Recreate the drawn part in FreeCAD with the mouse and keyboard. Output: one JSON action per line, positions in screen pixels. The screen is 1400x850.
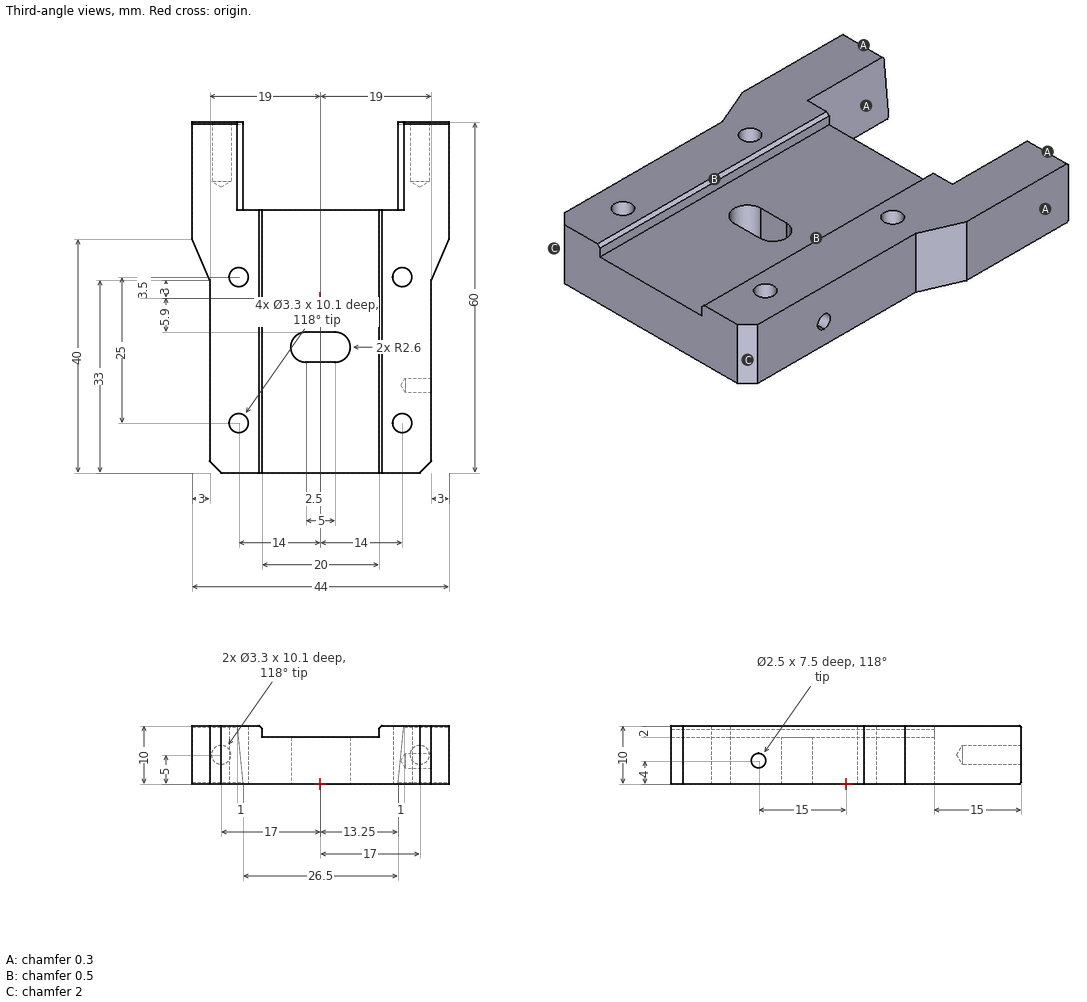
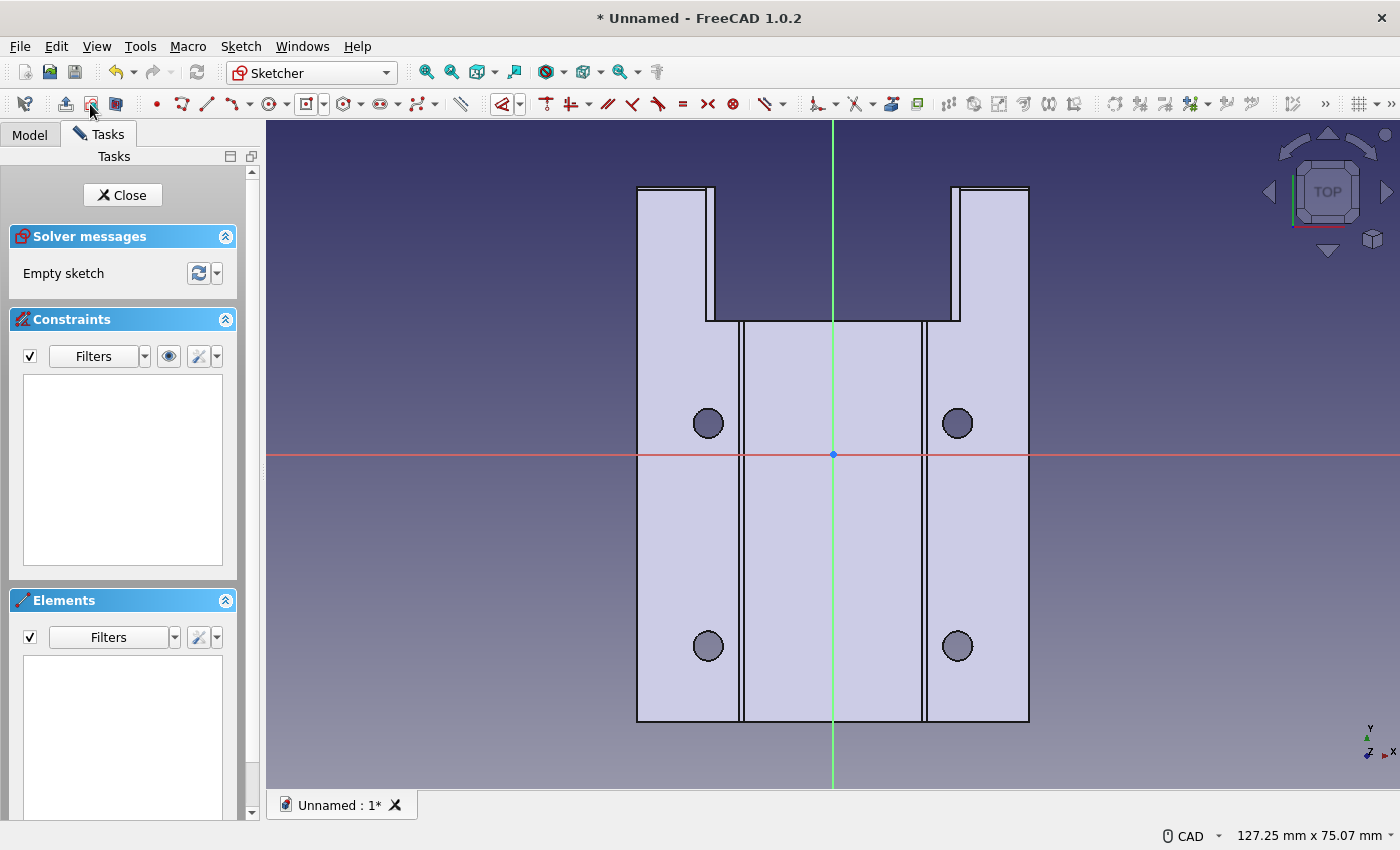
{"action": "left_click", "coordinate": [182, 104]}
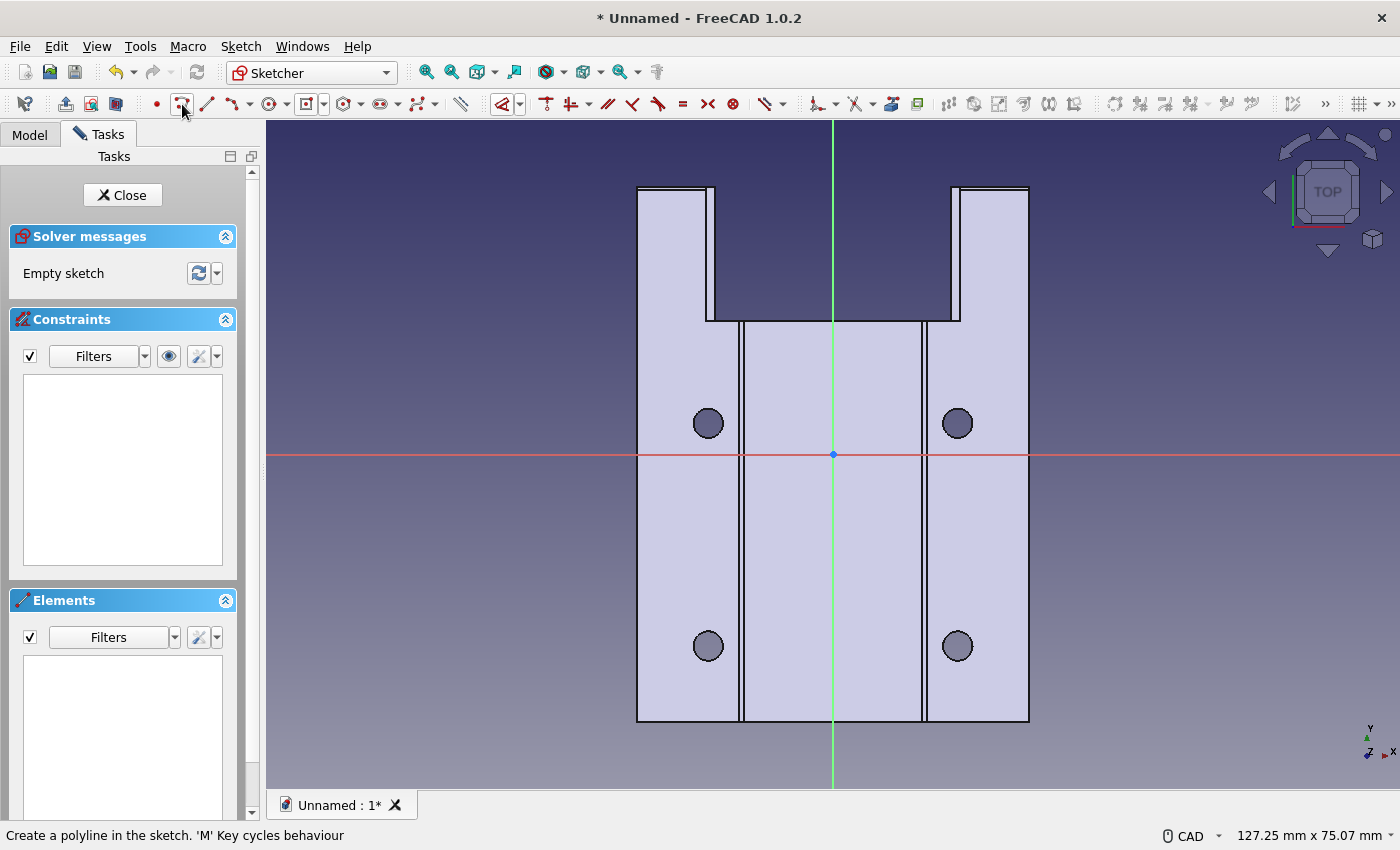
{"action": "left_click", "coordinate": [664, 428]}
{"action": "left_click", "coordinate": [637, 365]}
{"action": "left_click", "coordinate": [637, 722]}
{"action": "left_click", "coordinate": [664, 722]}
{"action": "left_click", "coordinate": [664, 429]}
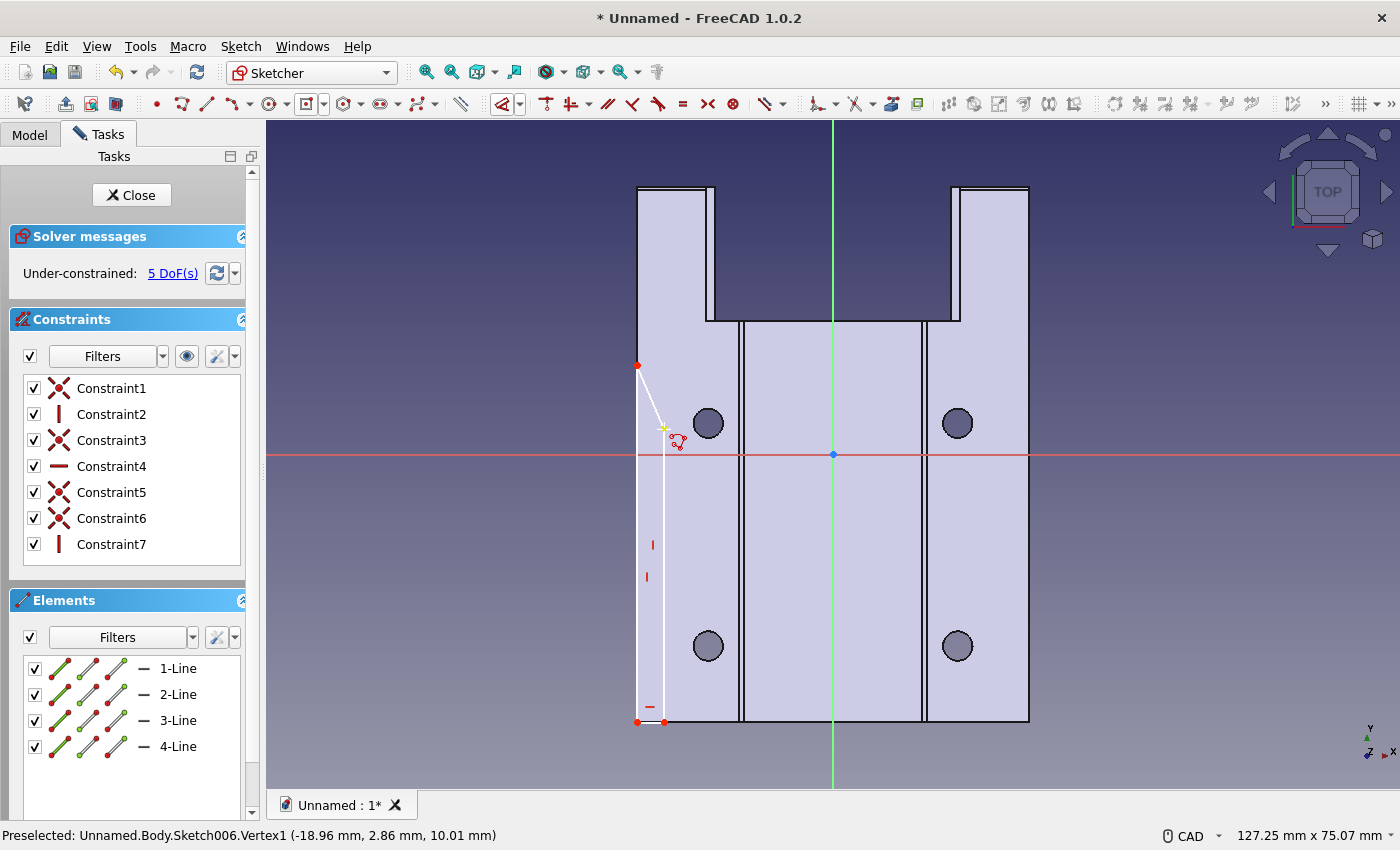
{"action": "left_click", "coordinate": [1002, 428]}
{"action": "left_click", "coordinate": [1002, 722]}
{"action": "left_click", "coordinate": [1029, 722]}
{"action": "left_click", "coordinate": [1029, 365]}
{"action": "left_click", "coordinate": [1002, 429]}
{"action": "key", "text": "Escape"}
{"action": "key", "text": "Escape"}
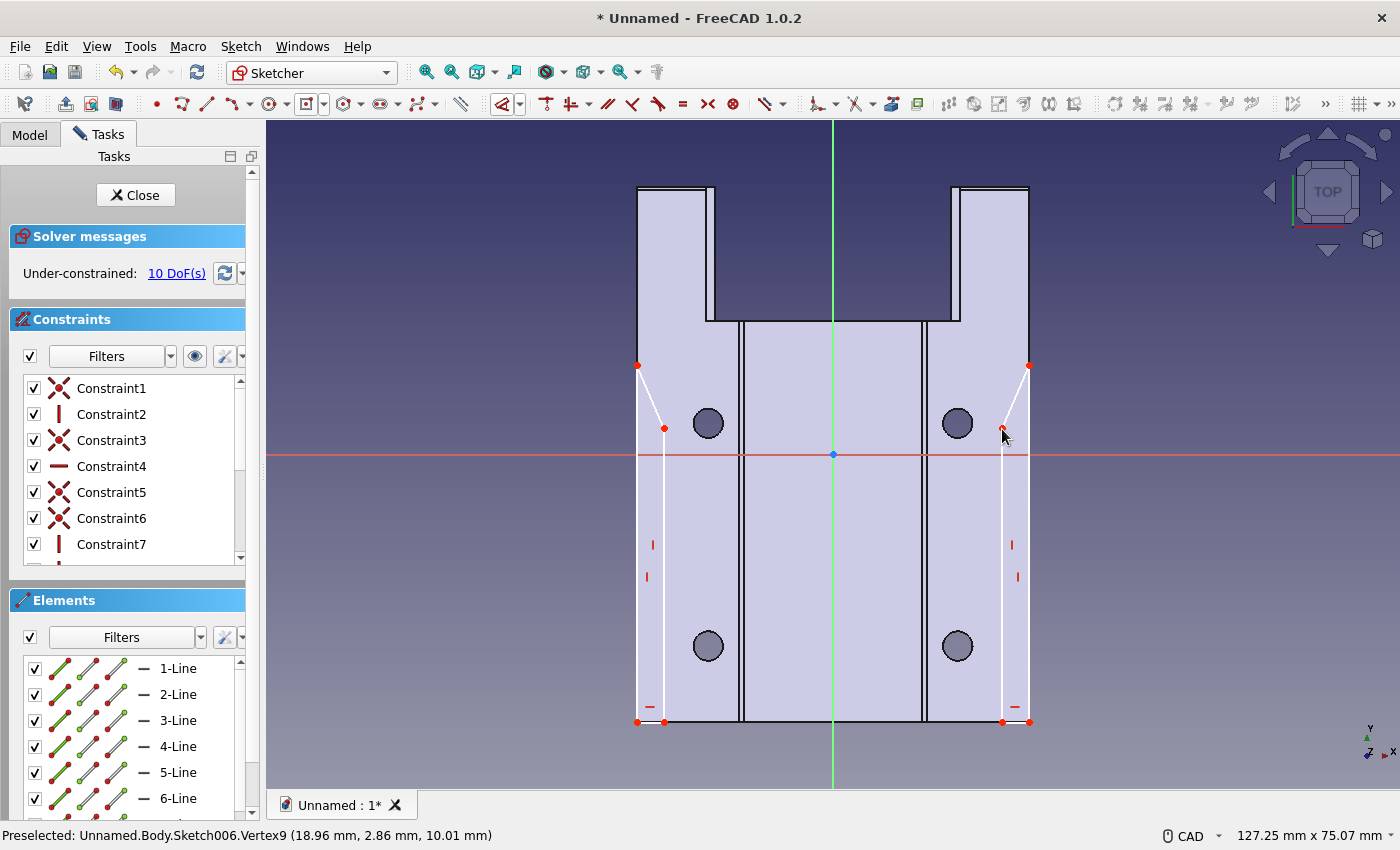
{"action": "scroll", "coordinate": [648, 723], "scroll_direction": "up", "scroll_amount": 2}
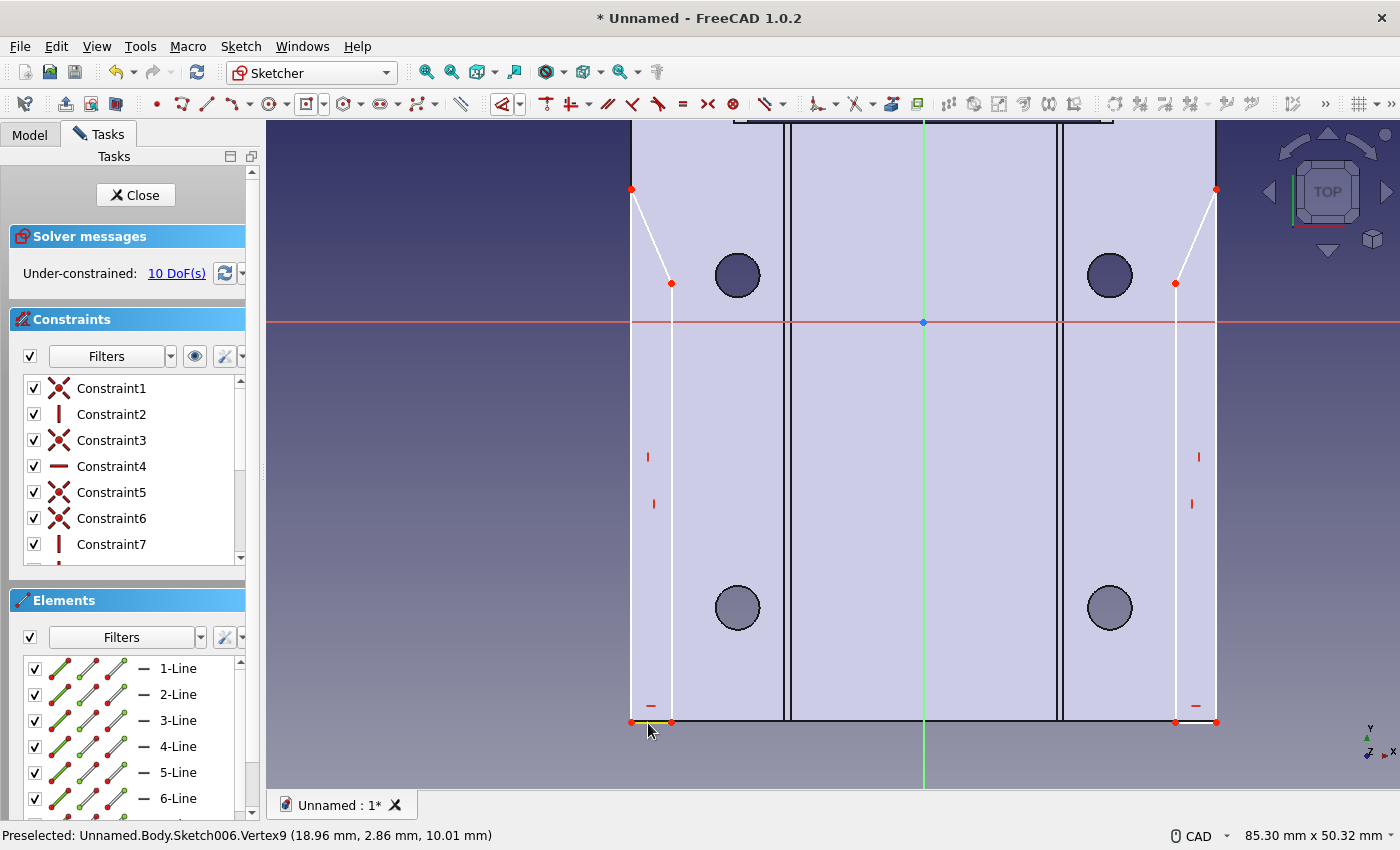
{"action": "left_click", "coordinate": [648, 723]}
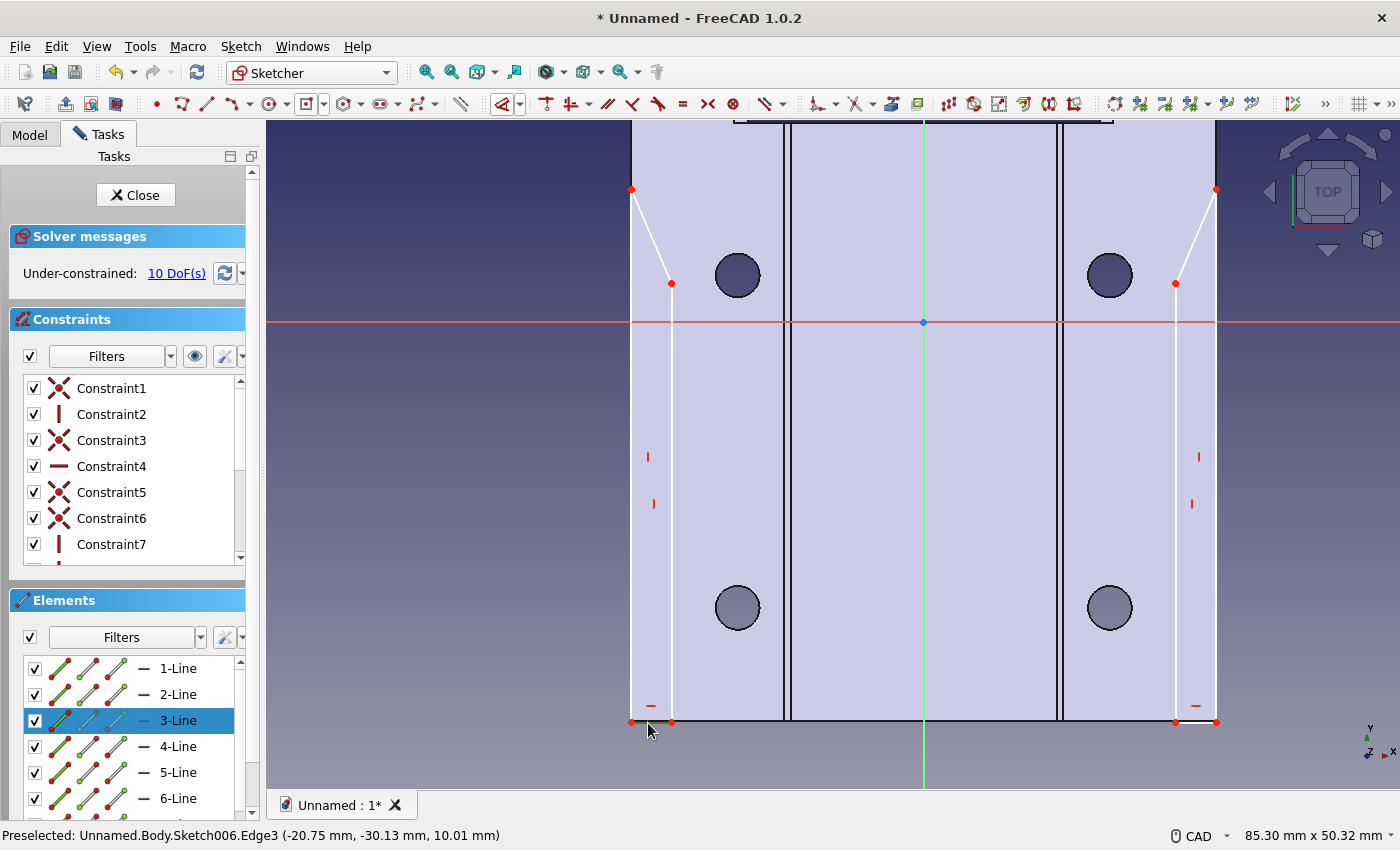
{"action": "key", "text": "l"}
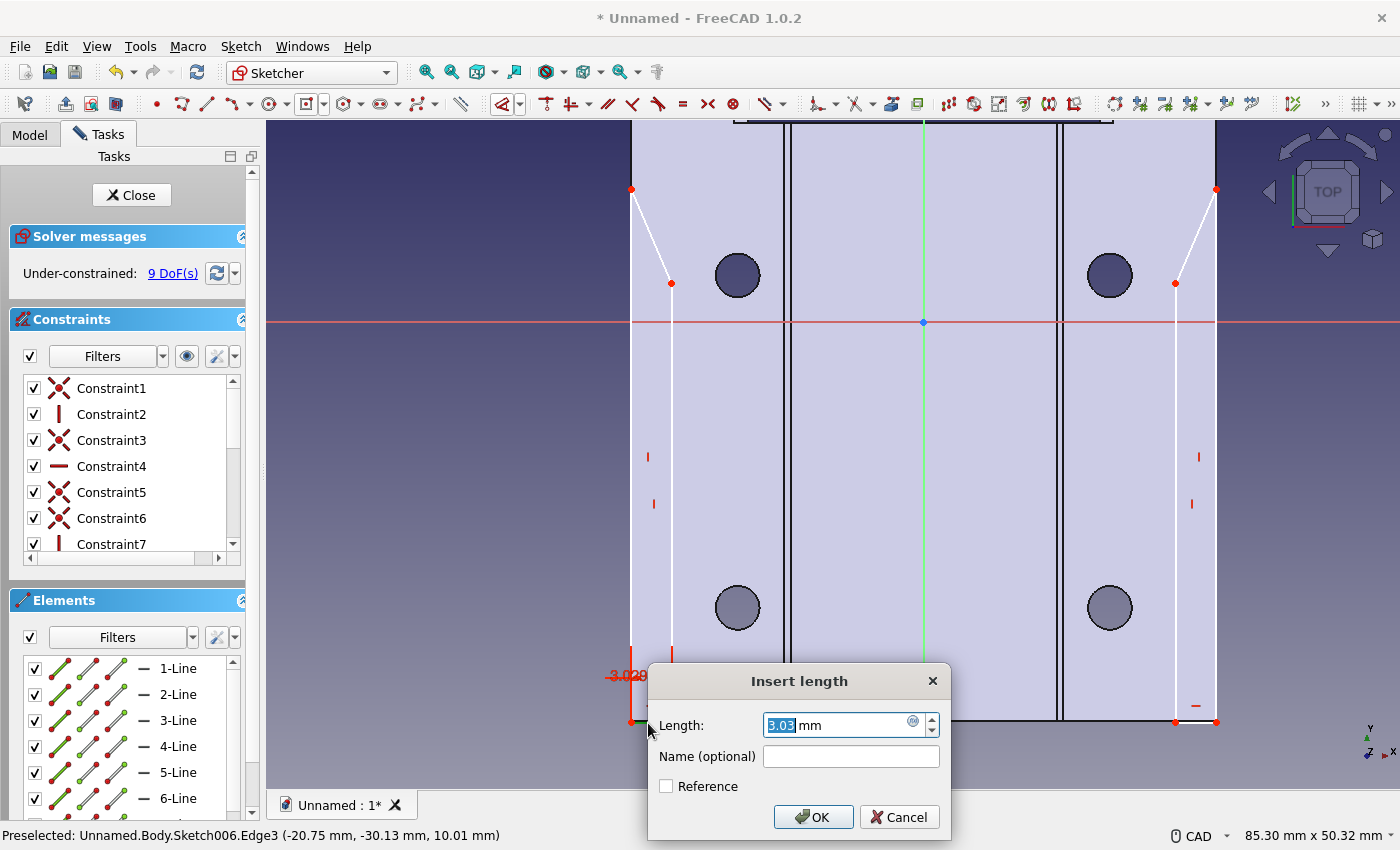
{"action": "type", "text": "3"}
{"action": "key", "text": "Return"}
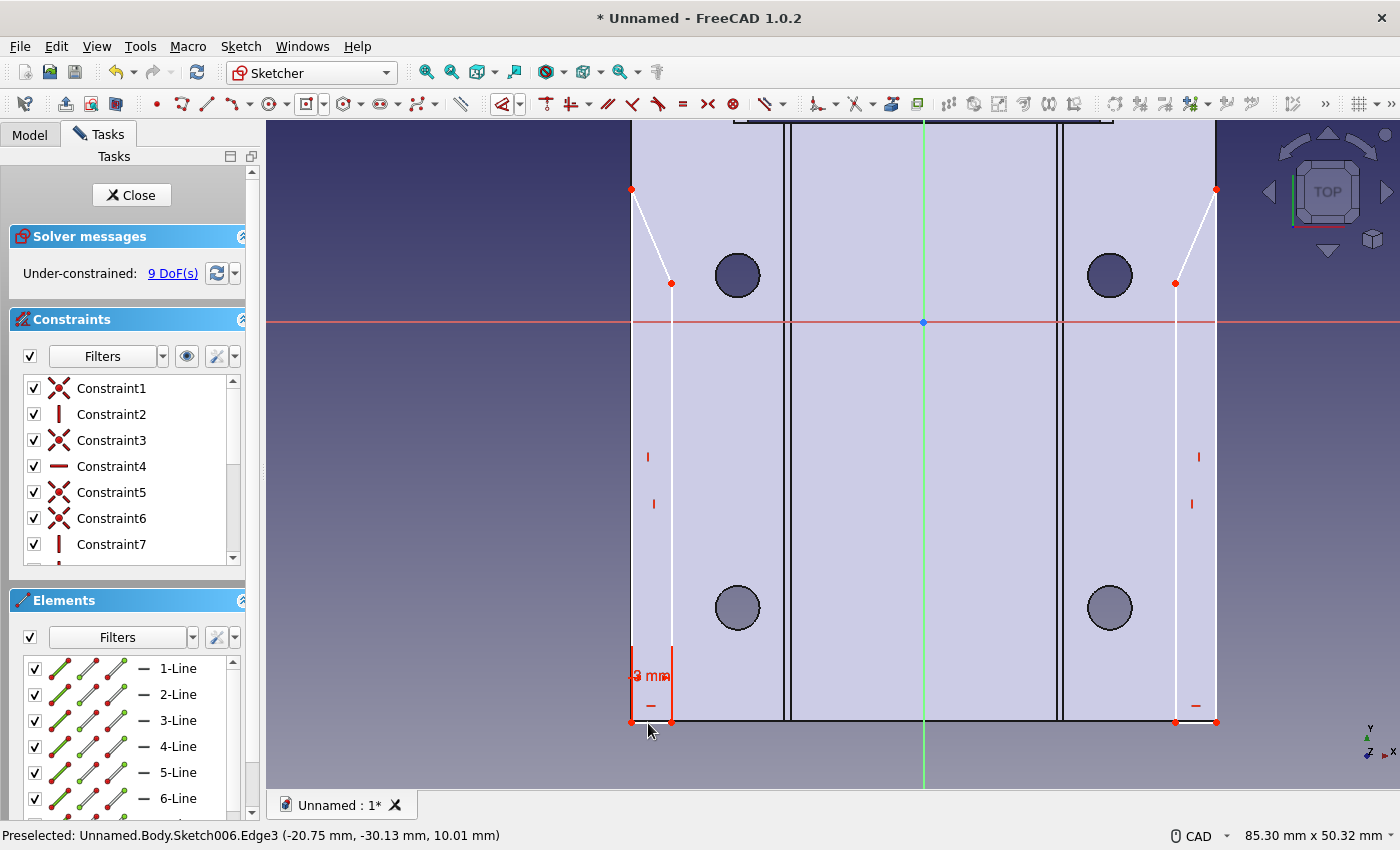
{"action": "left_click", "coordinate": [1188, 723]}